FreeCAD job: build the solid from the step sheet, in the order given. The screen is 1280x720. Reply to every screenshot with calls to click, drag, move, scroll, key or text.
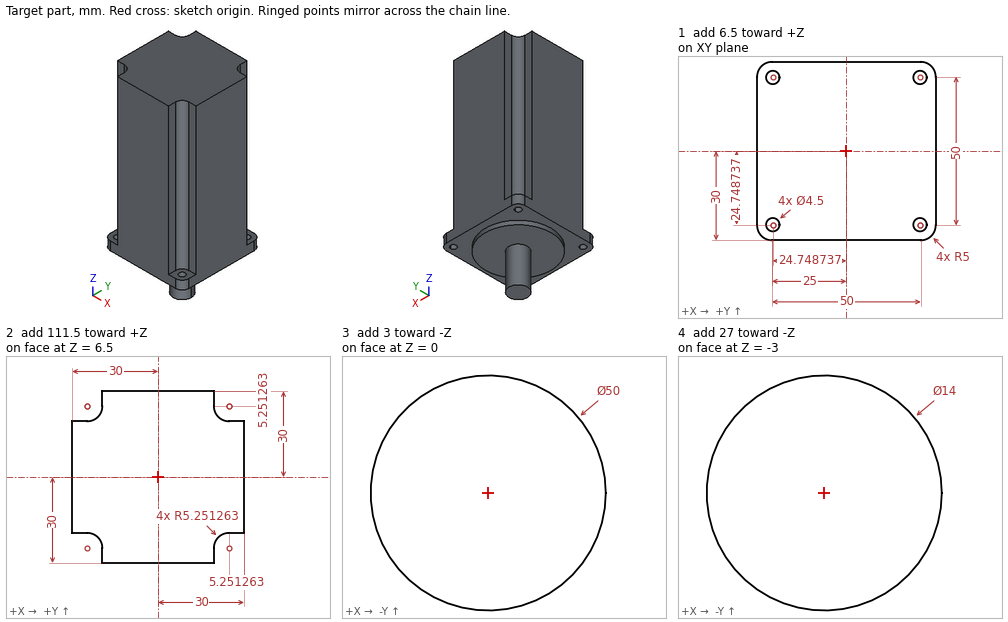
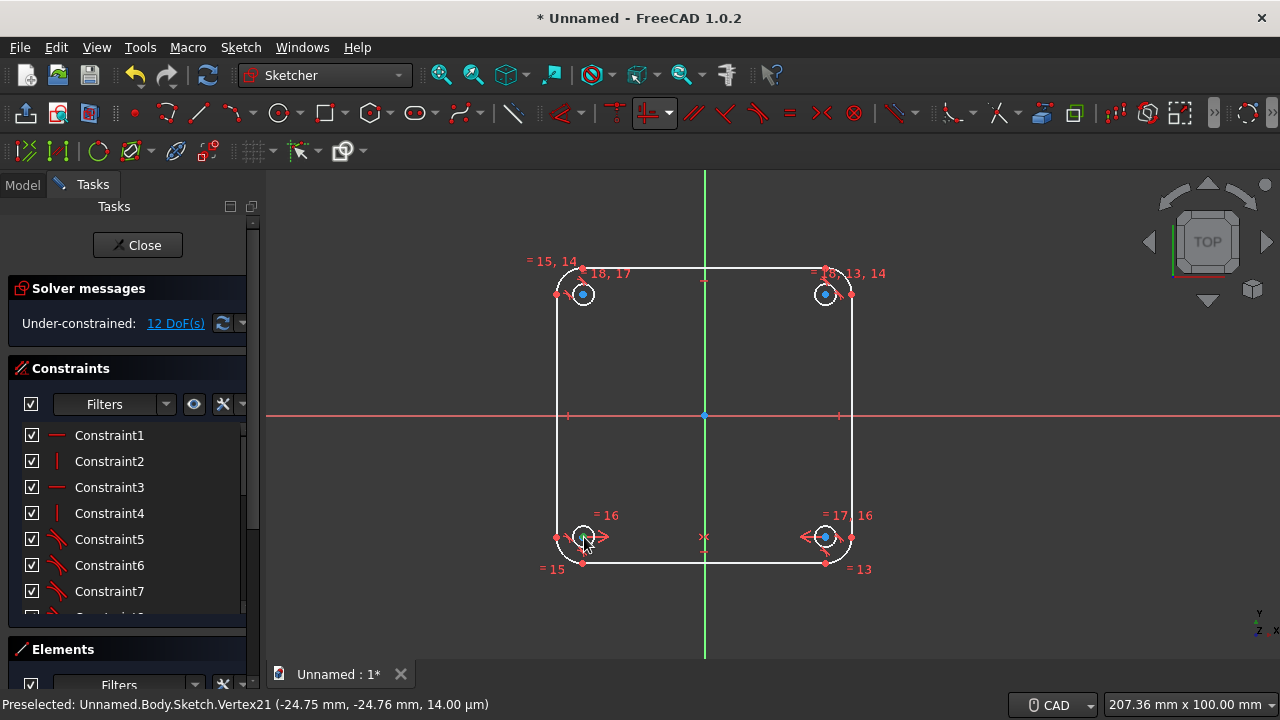
scroll(584, 295, up, 12)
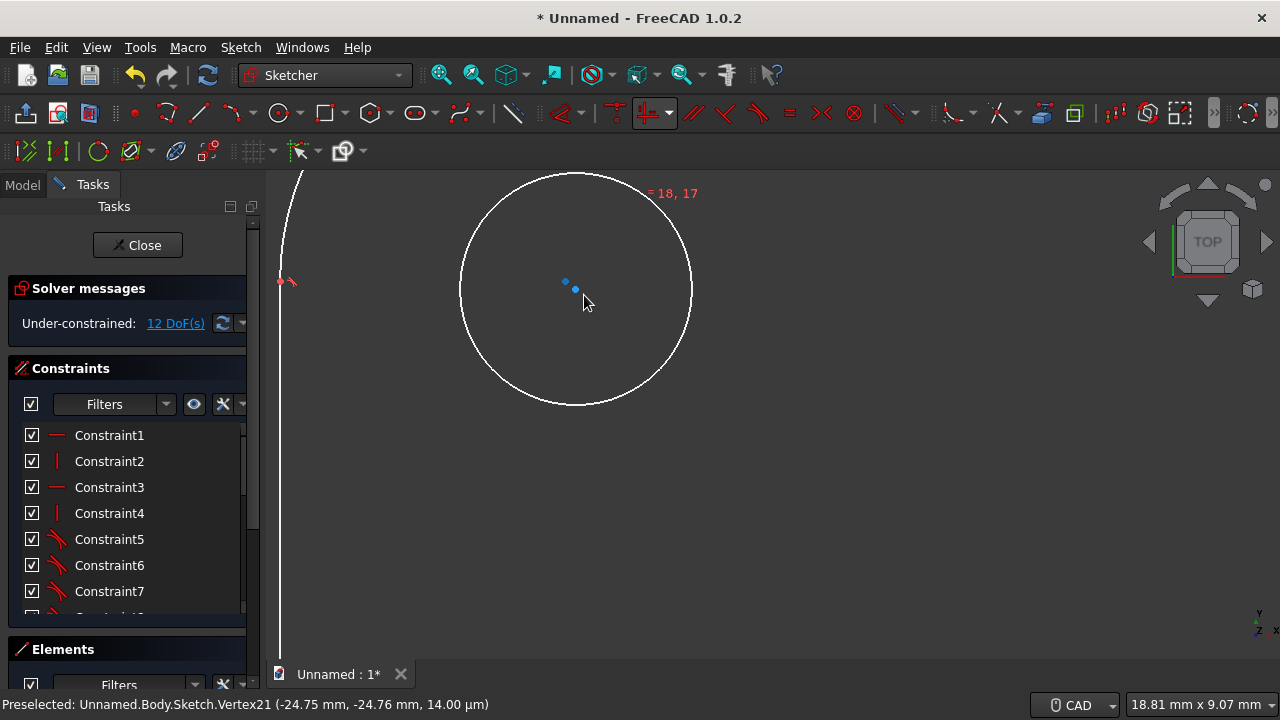
click(576, 289)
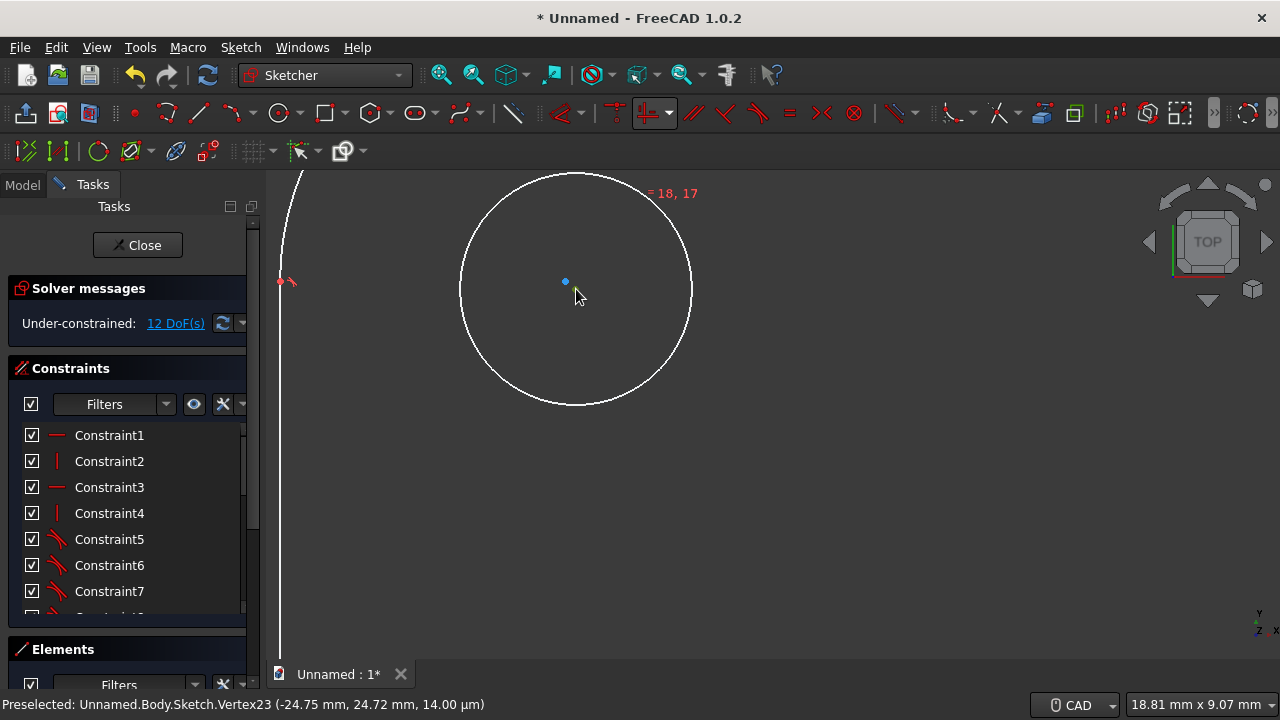
scroll(584, 294, down, 12)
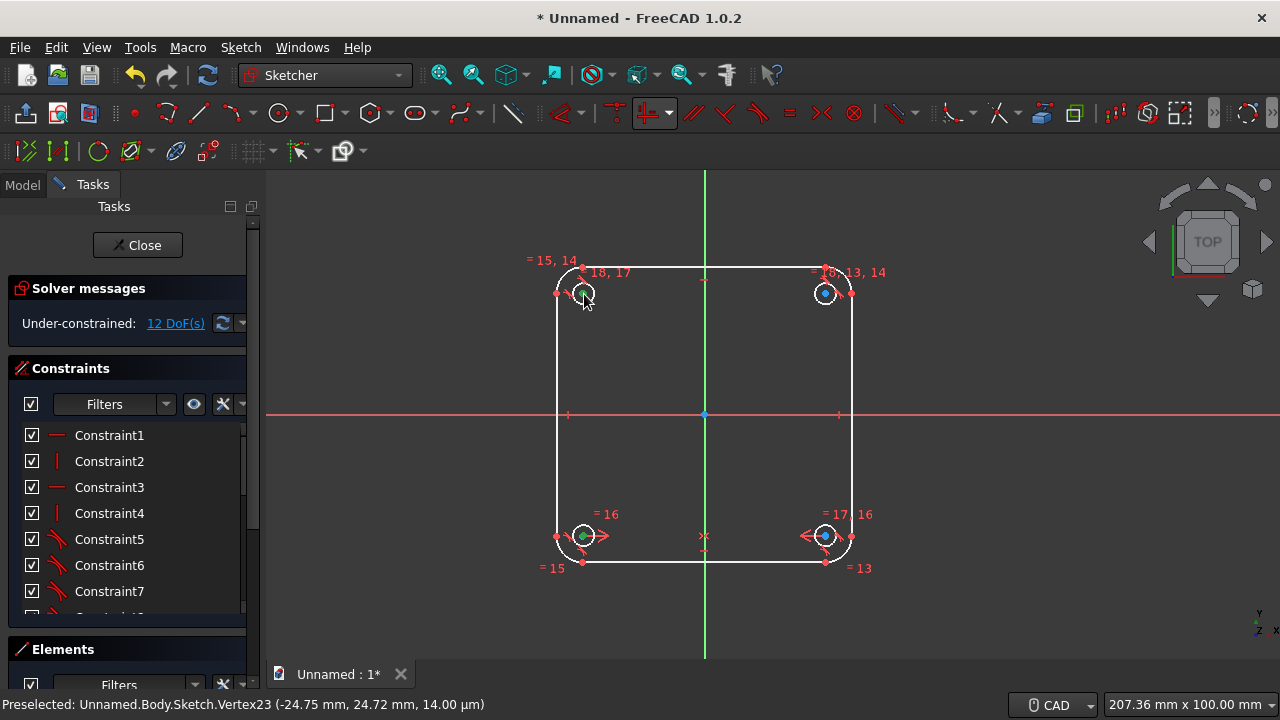
click(353, 415)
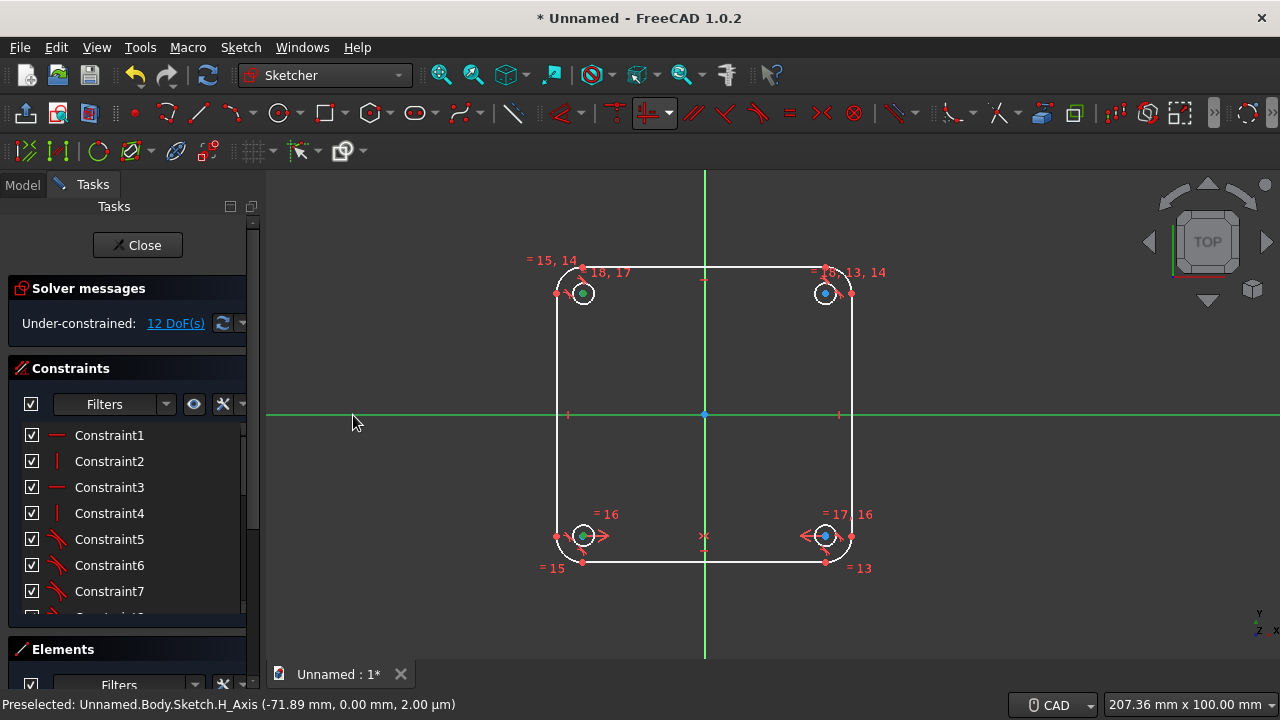
key(s)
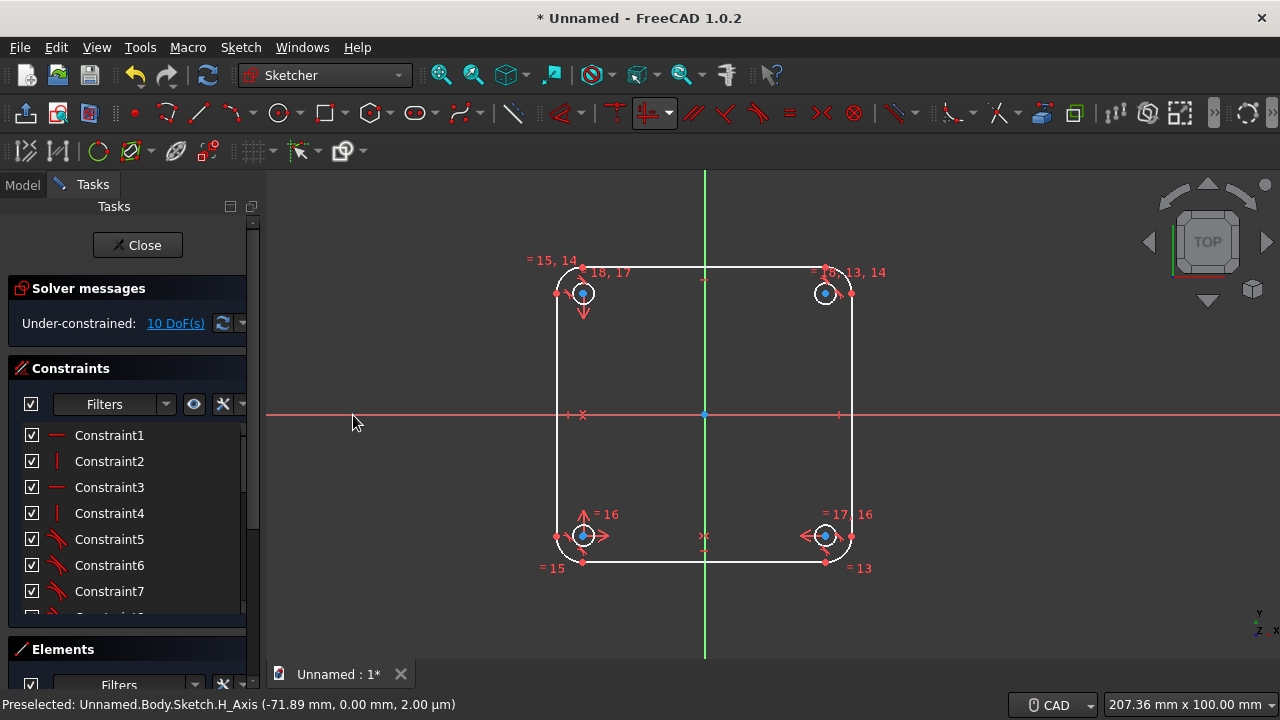
scroll(826, 536, up, 14)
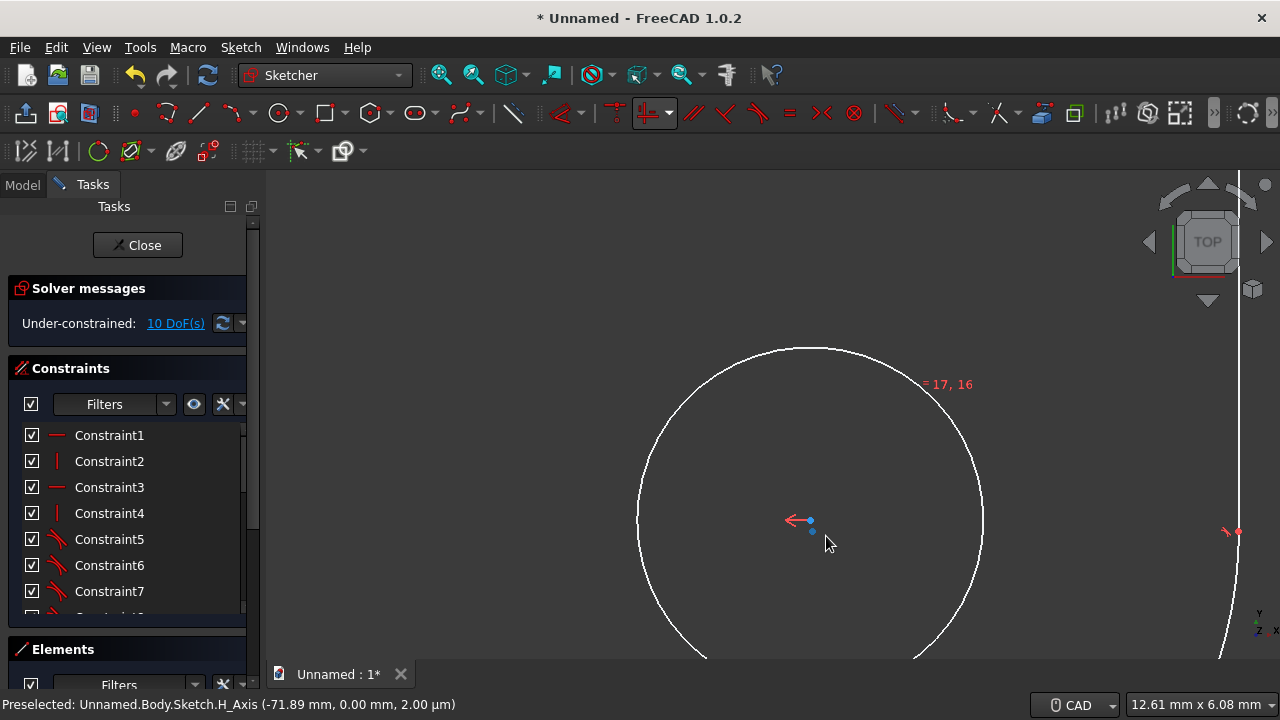
click(810, 520)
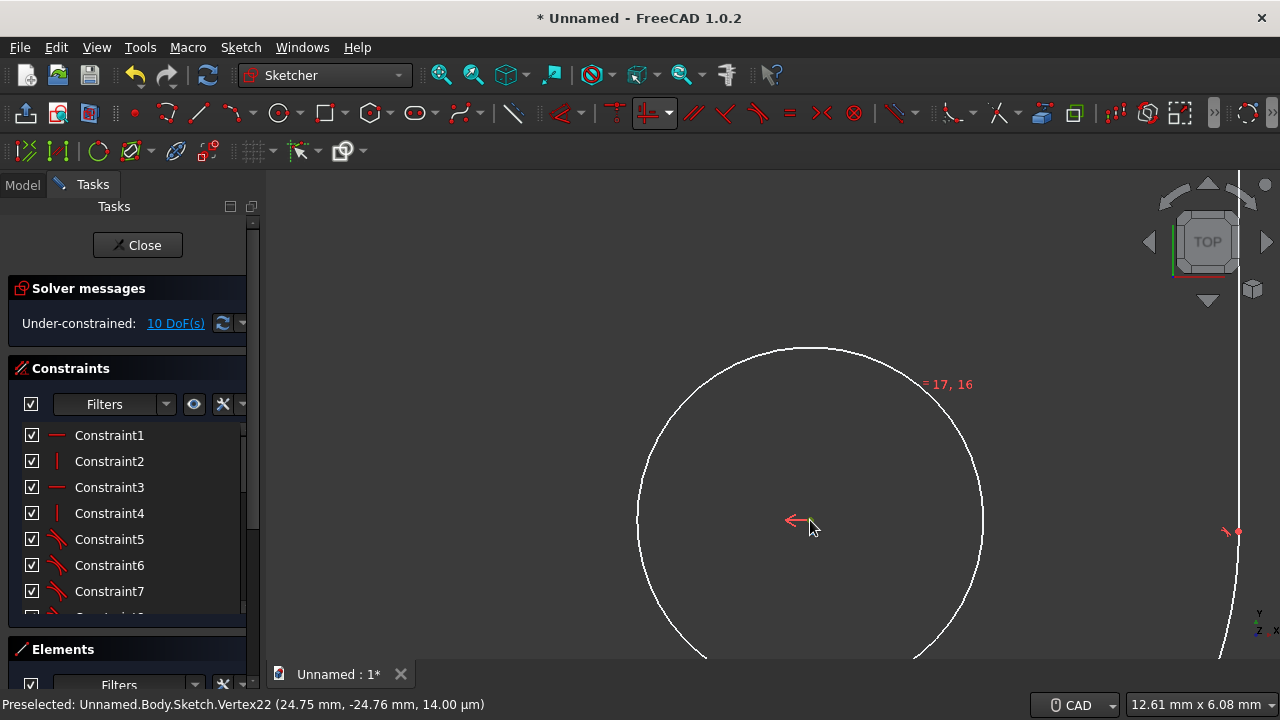
scroll(826, 537, down, 14)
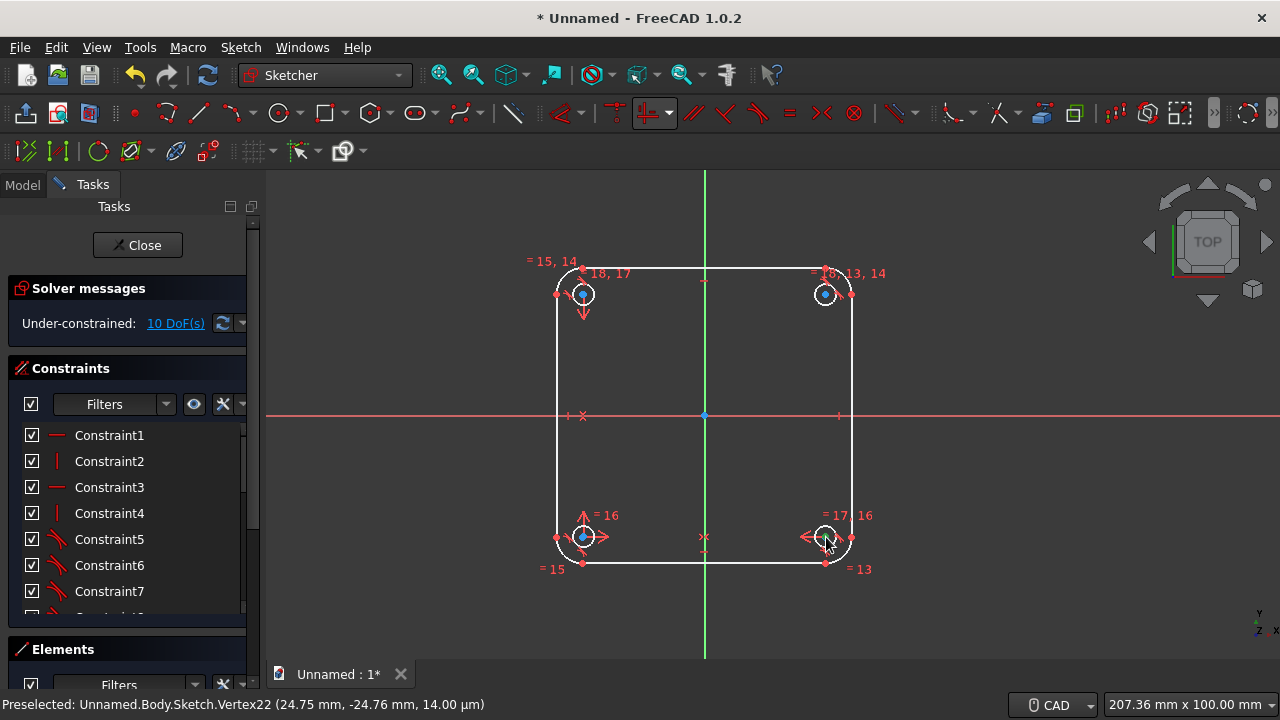
scroll(826, 295, up, 14)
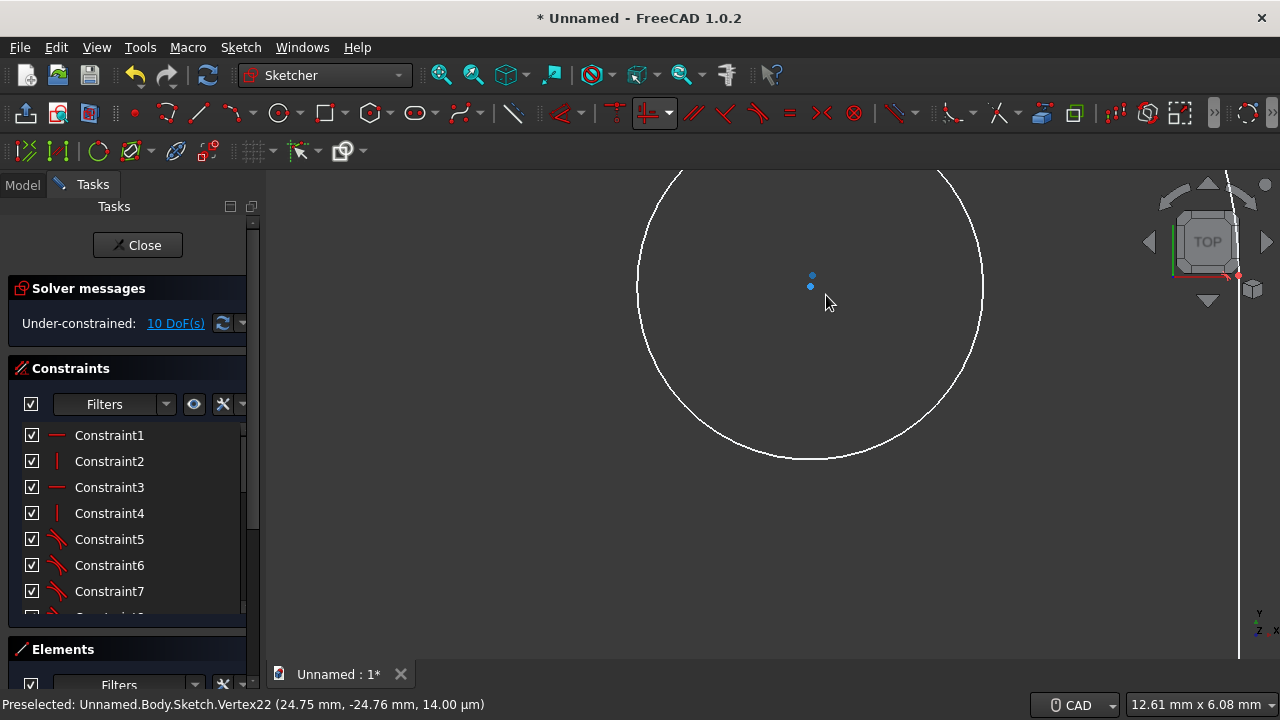
click(810, 287)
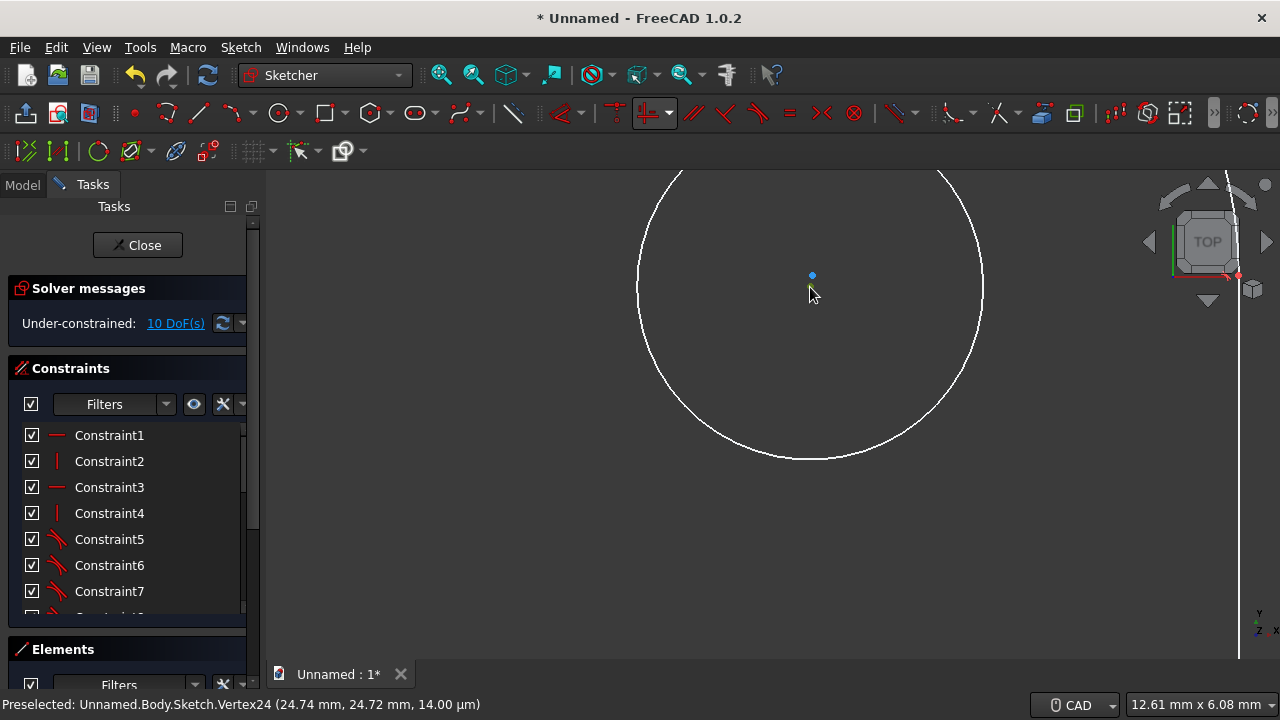
scroll(826, 294, down, 14)